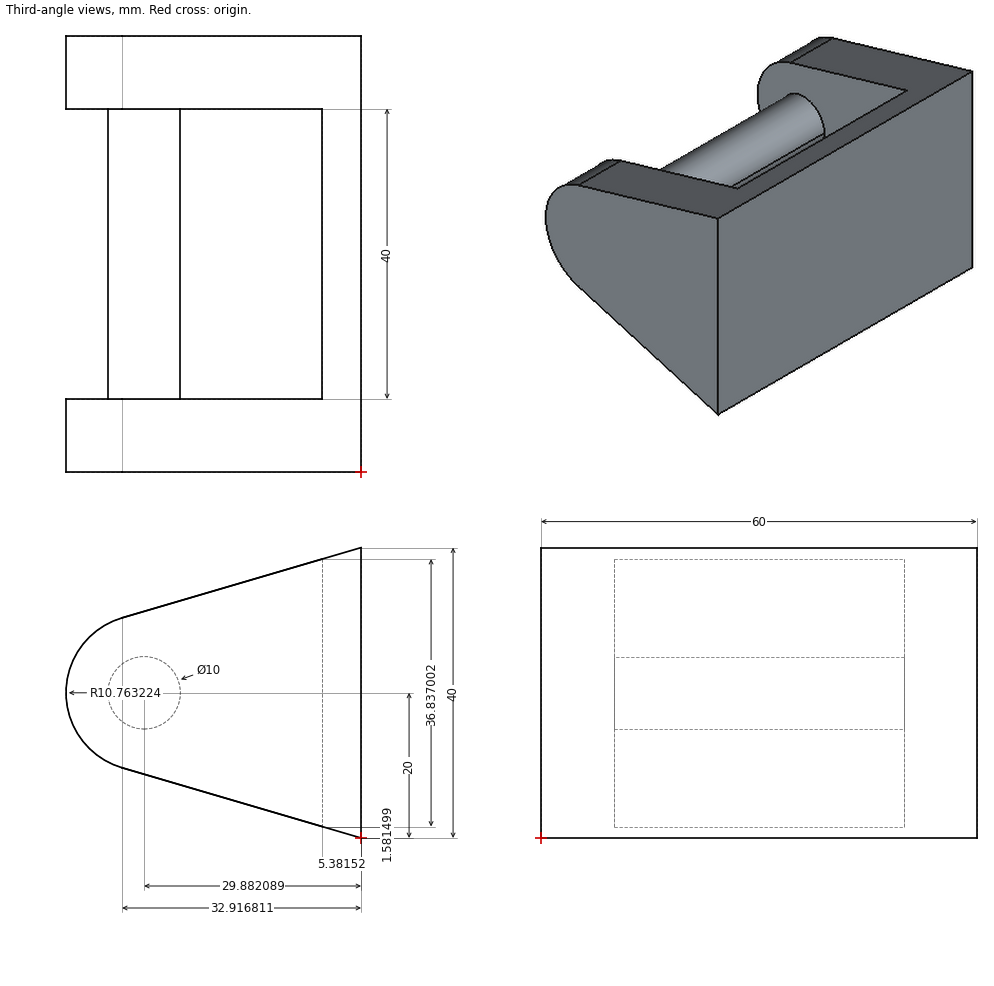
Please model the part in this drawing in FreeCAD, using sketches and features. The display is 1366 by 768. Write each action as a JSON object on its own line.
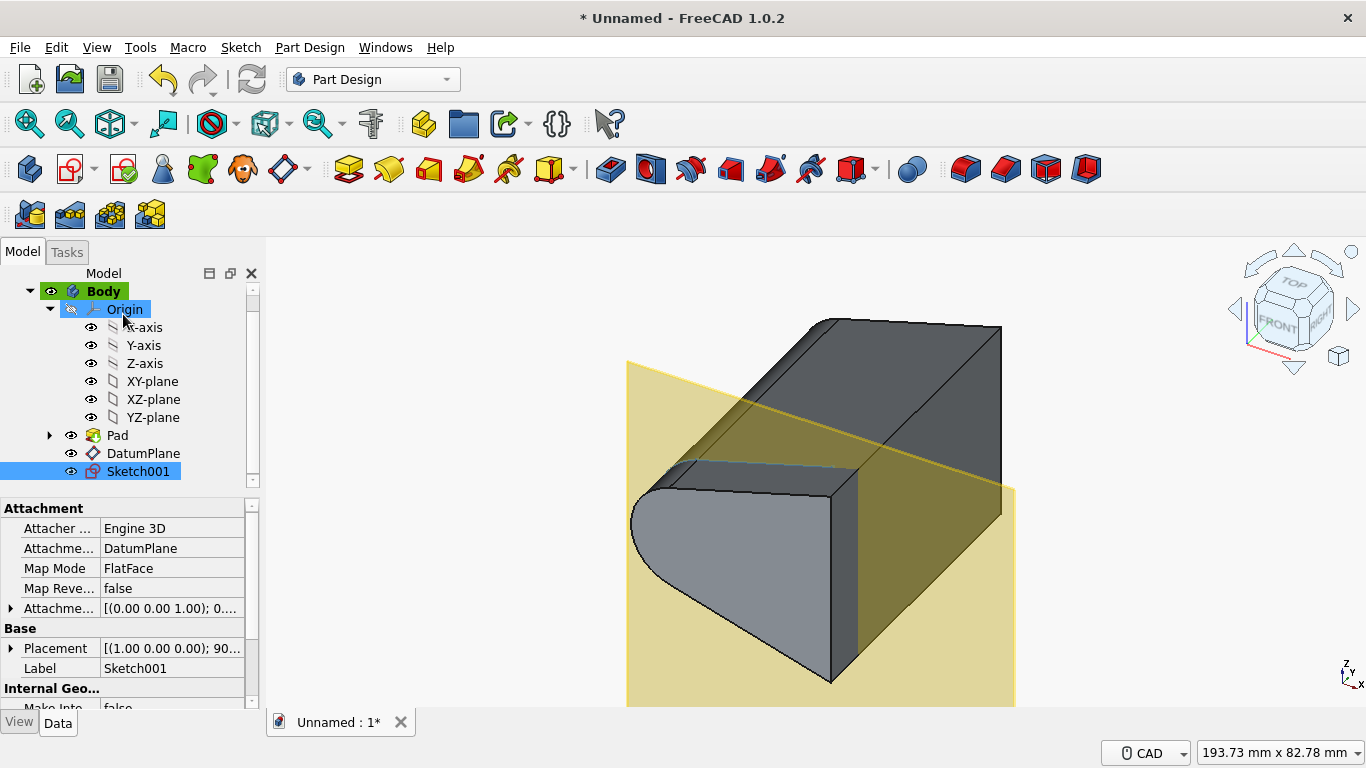
{"action": "left_click", "coordinate": [612, 170]}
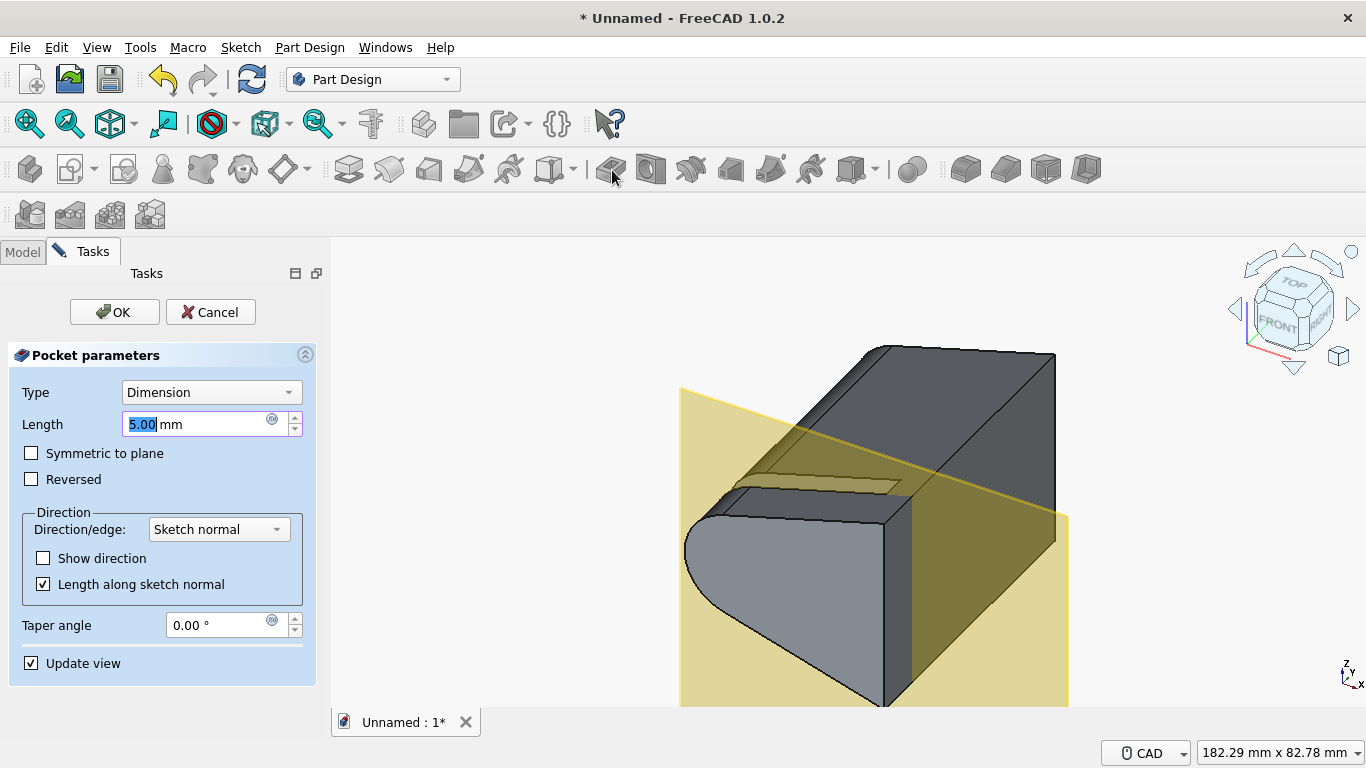
{"action": "type", "text": "40"}
{"action": "key", "text": "Tab"}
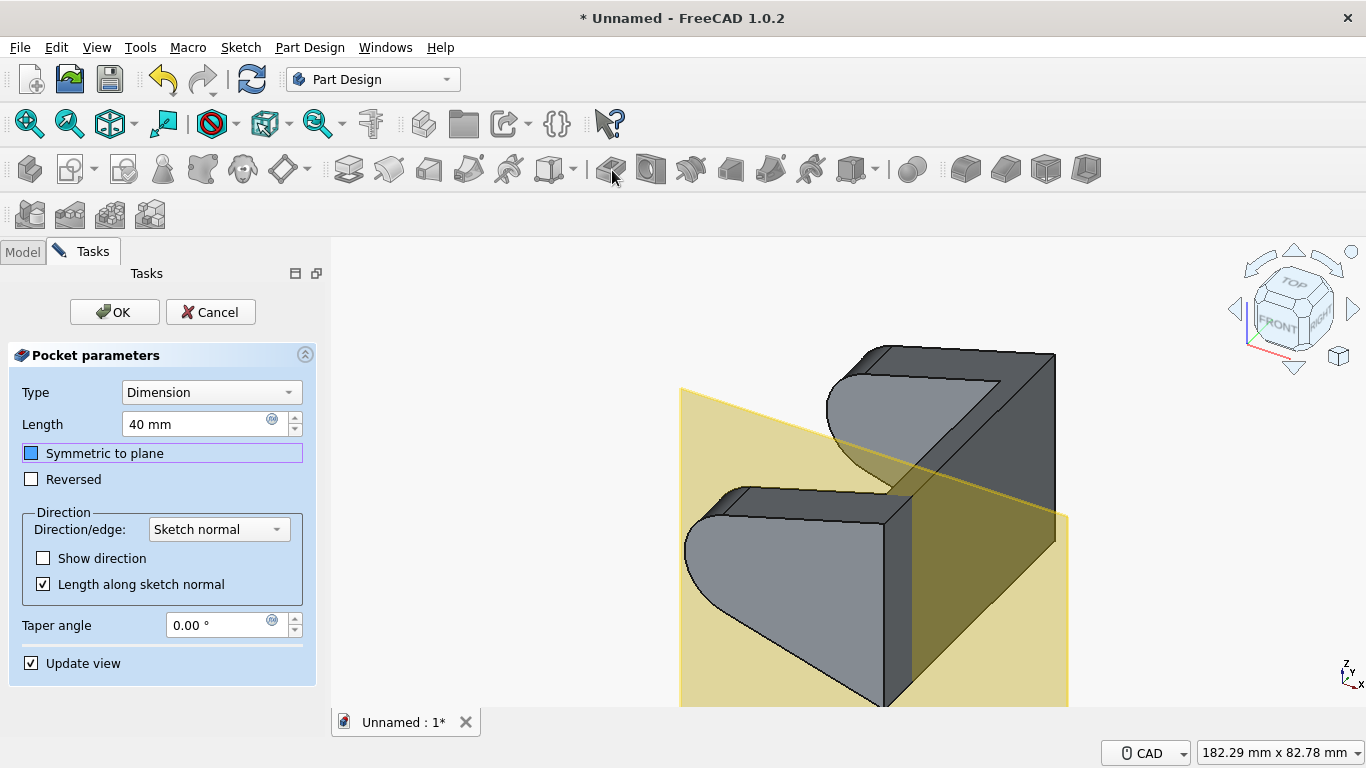
{"action": "left_click", "coordinate": [115, 312]}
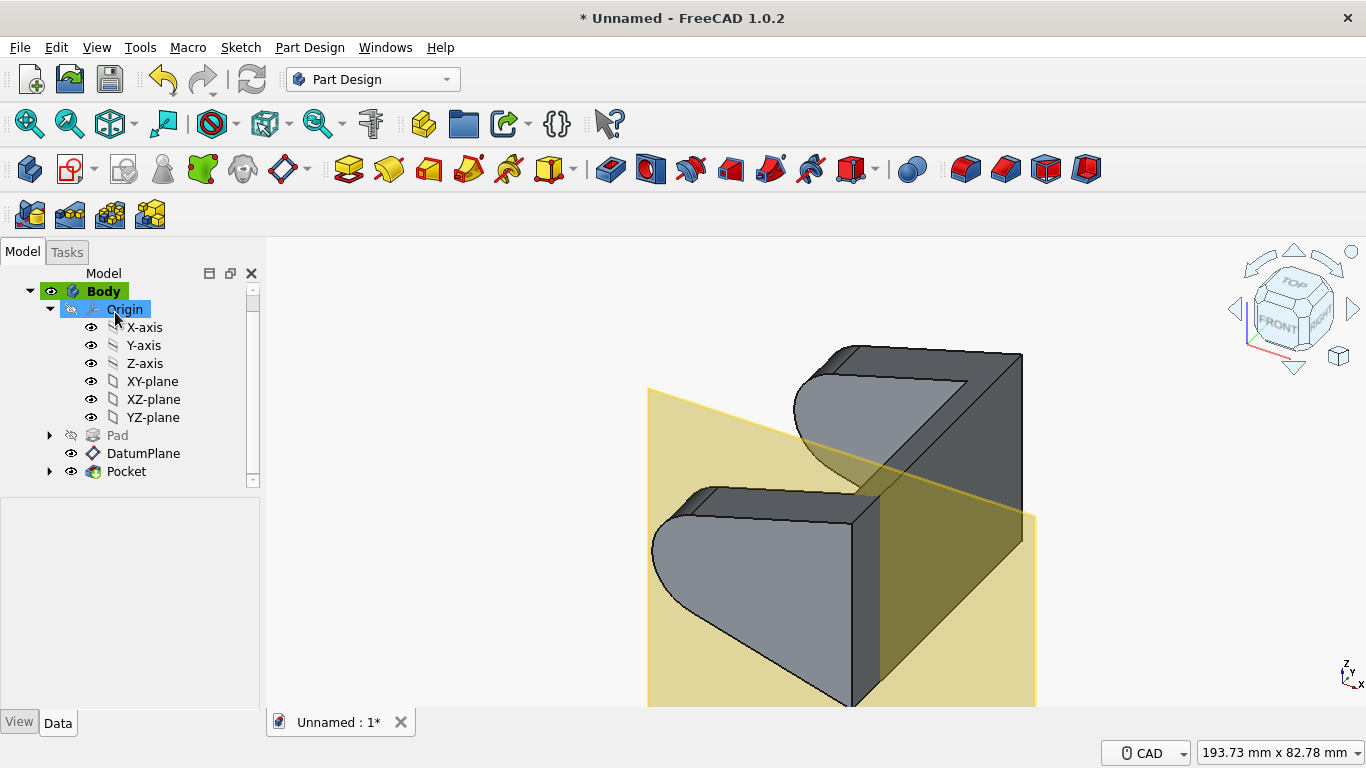
{"action": "left_click", "coordinate": [116, 453]}
{"action": "key", "text": "space"}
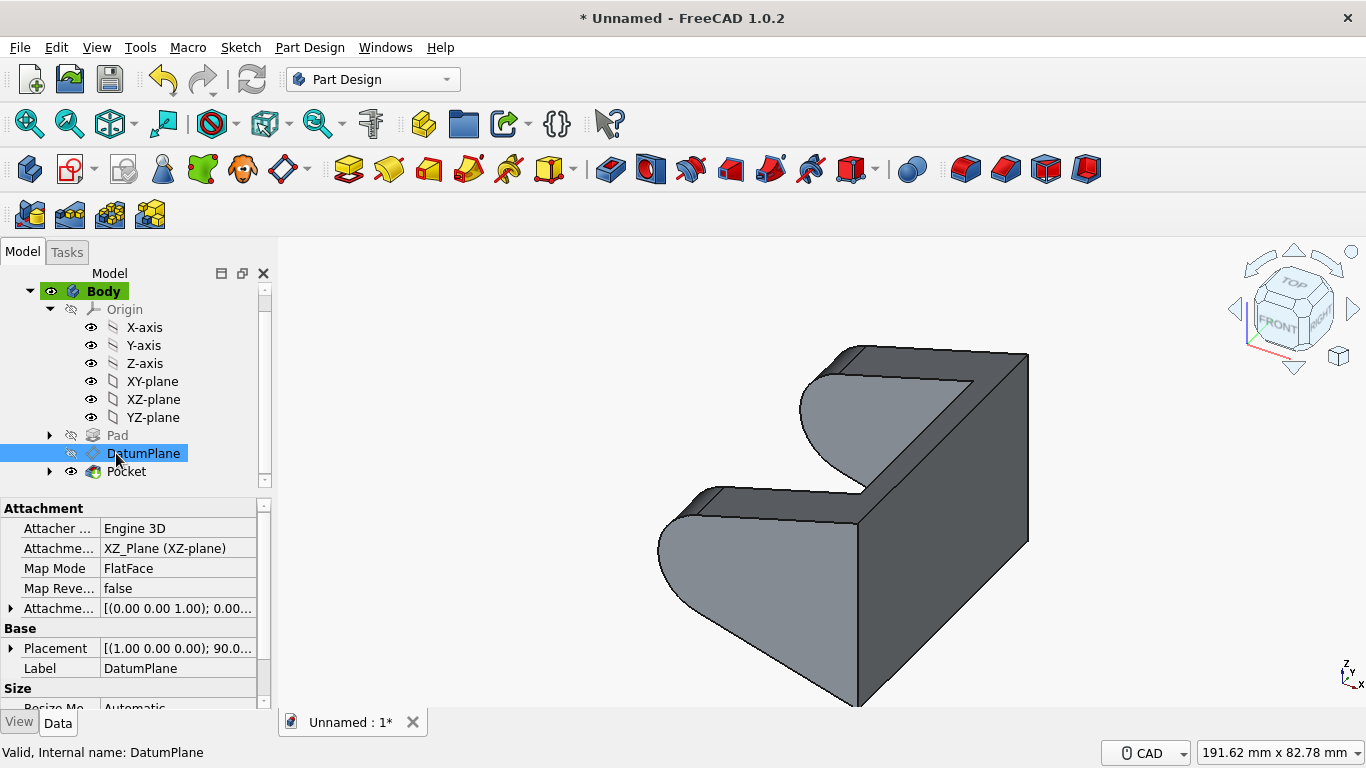
{"action": "left_click", "coordinate": [30, 124]}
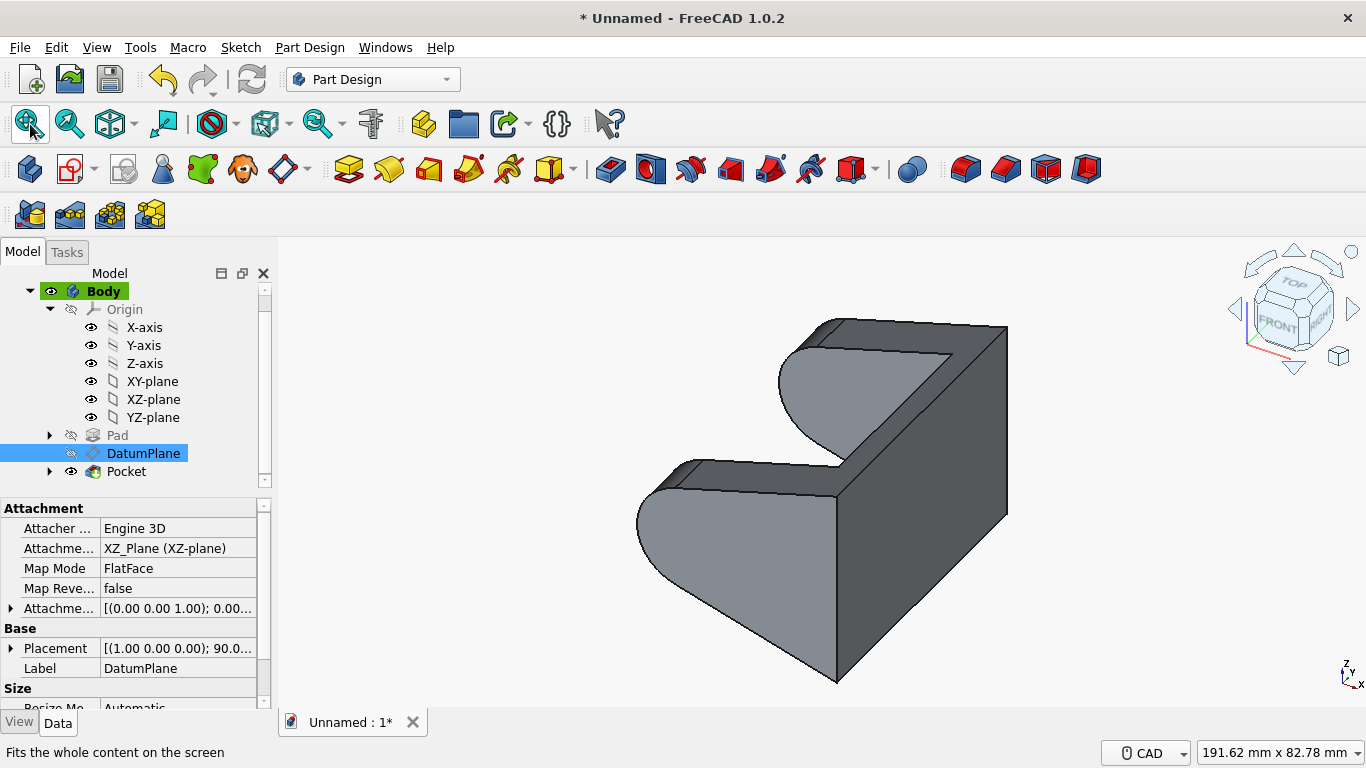
{"action": "left_click", "coordinate": [136, 399]}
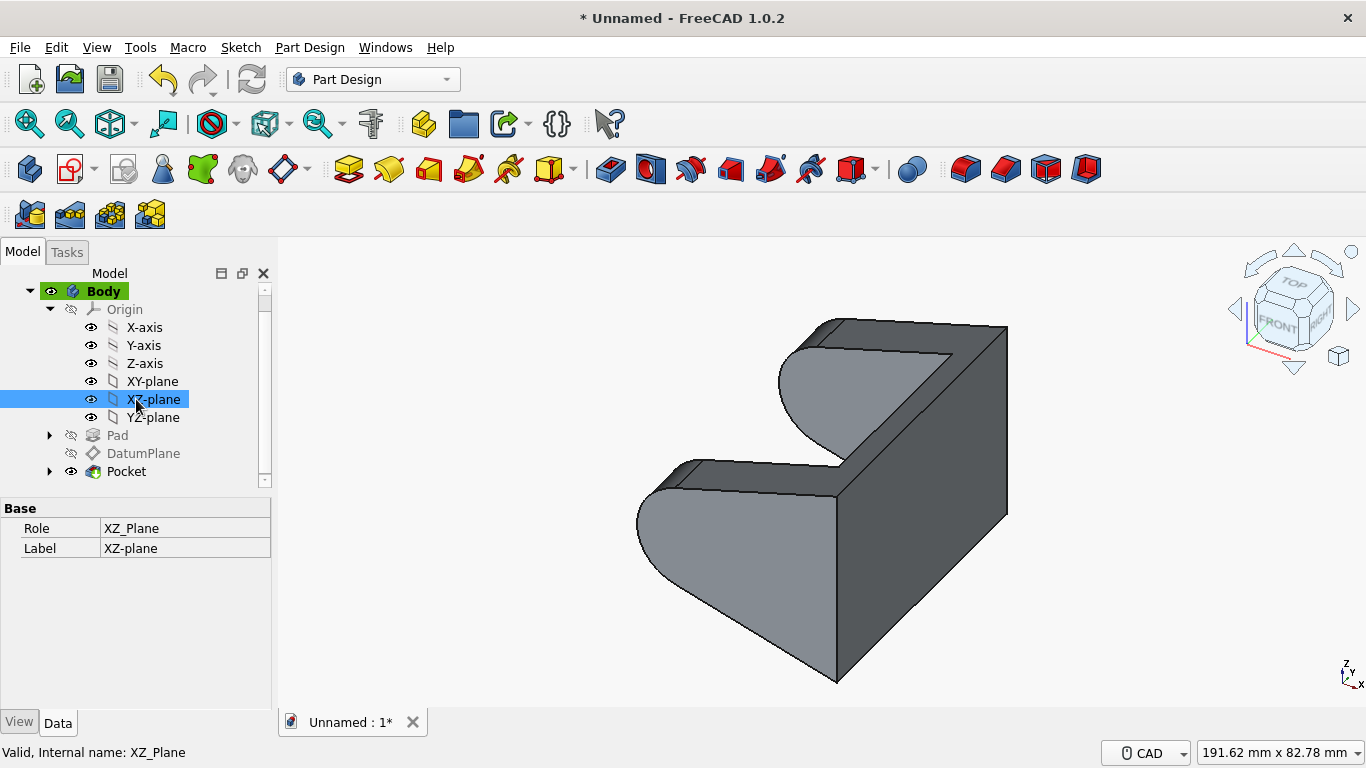
{"action": "left_click", "coordinate": [284, 170]}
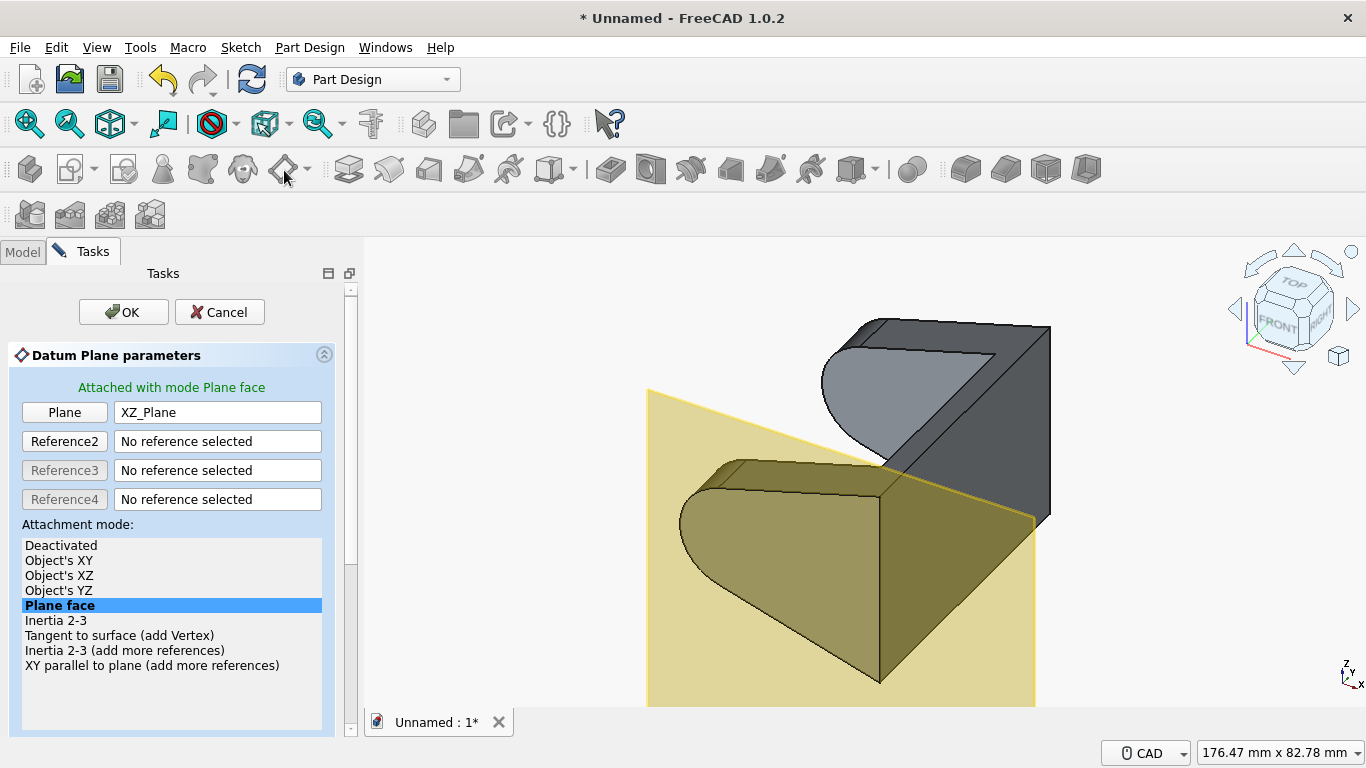
{"action": "scroll", "coordinate": [351, 510], "scroll_direction": "down", "scroll_amount": 3}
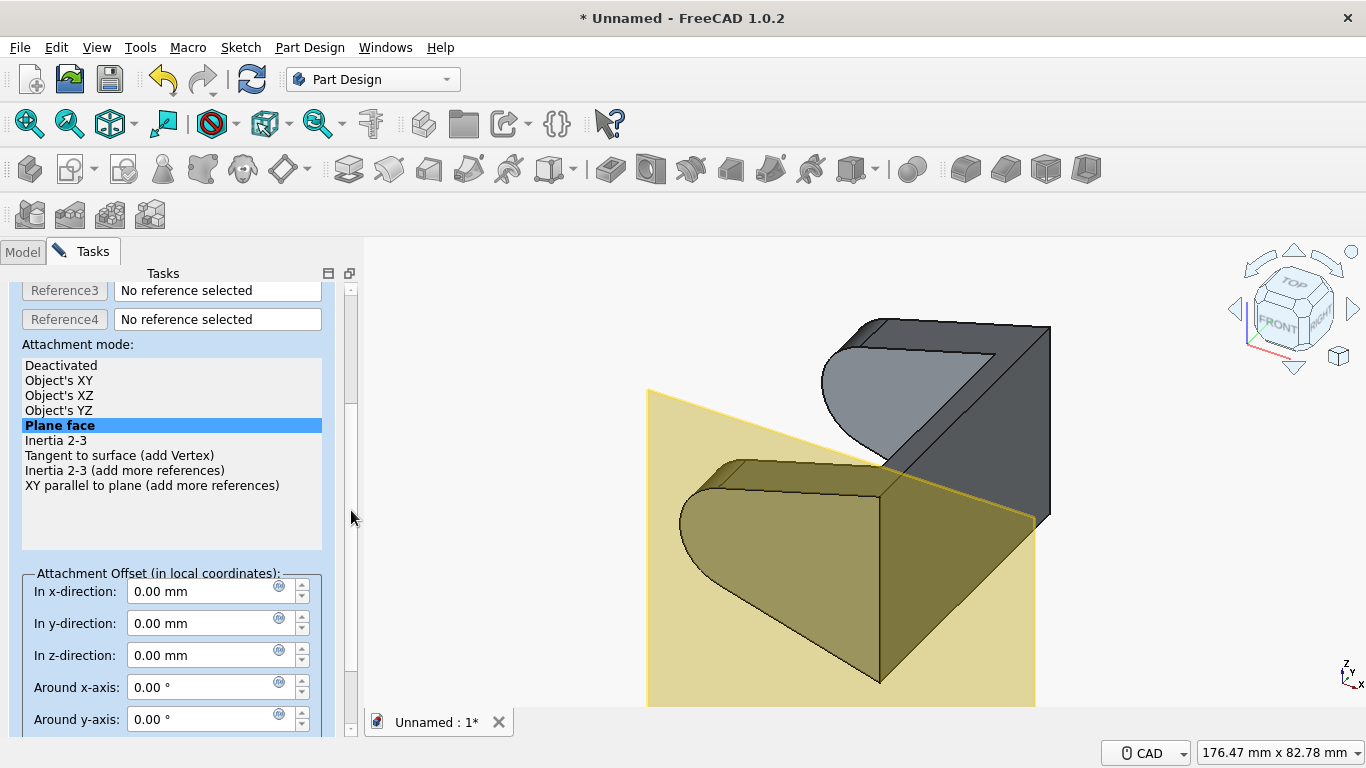
{"action": "triple_click", "coordinate": [210, 655]}